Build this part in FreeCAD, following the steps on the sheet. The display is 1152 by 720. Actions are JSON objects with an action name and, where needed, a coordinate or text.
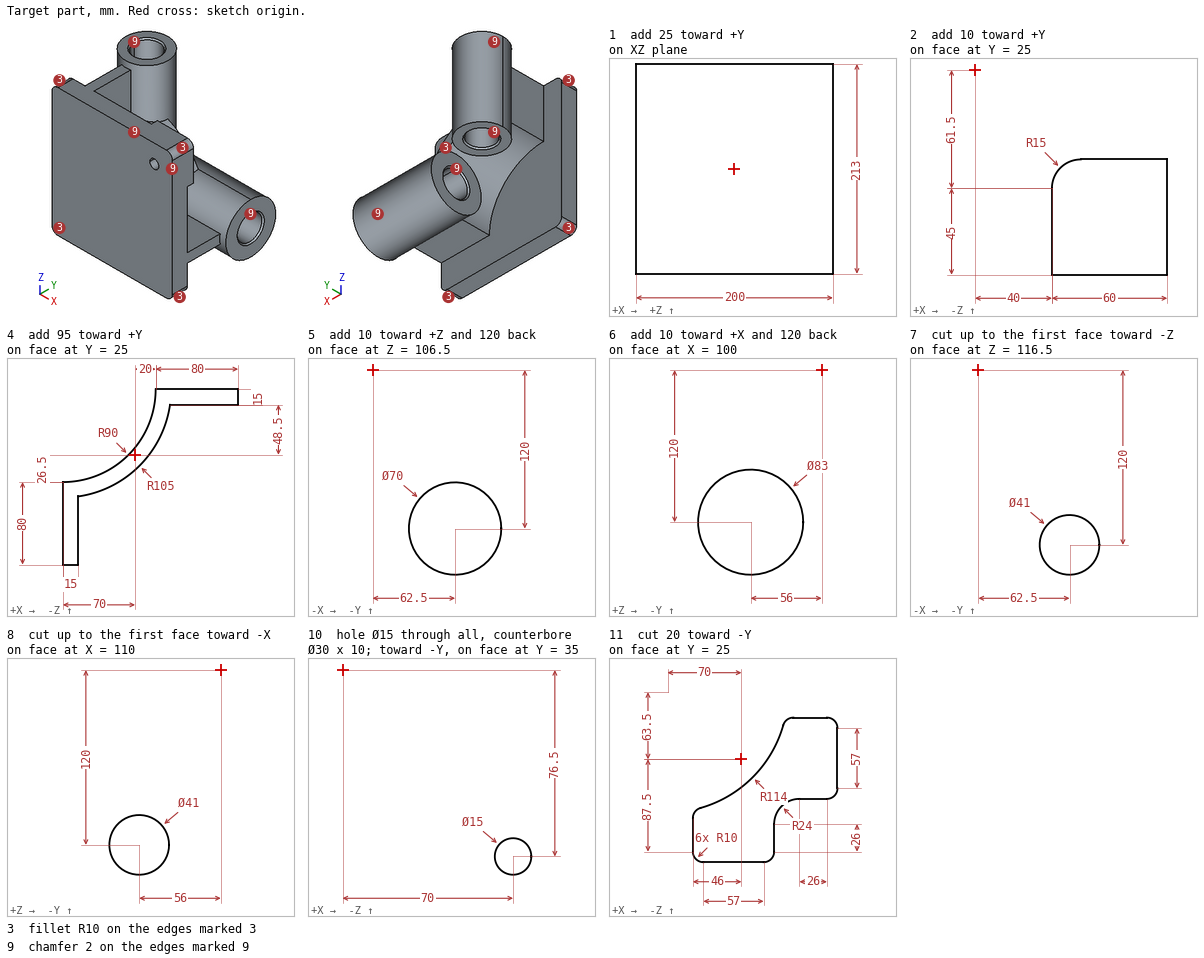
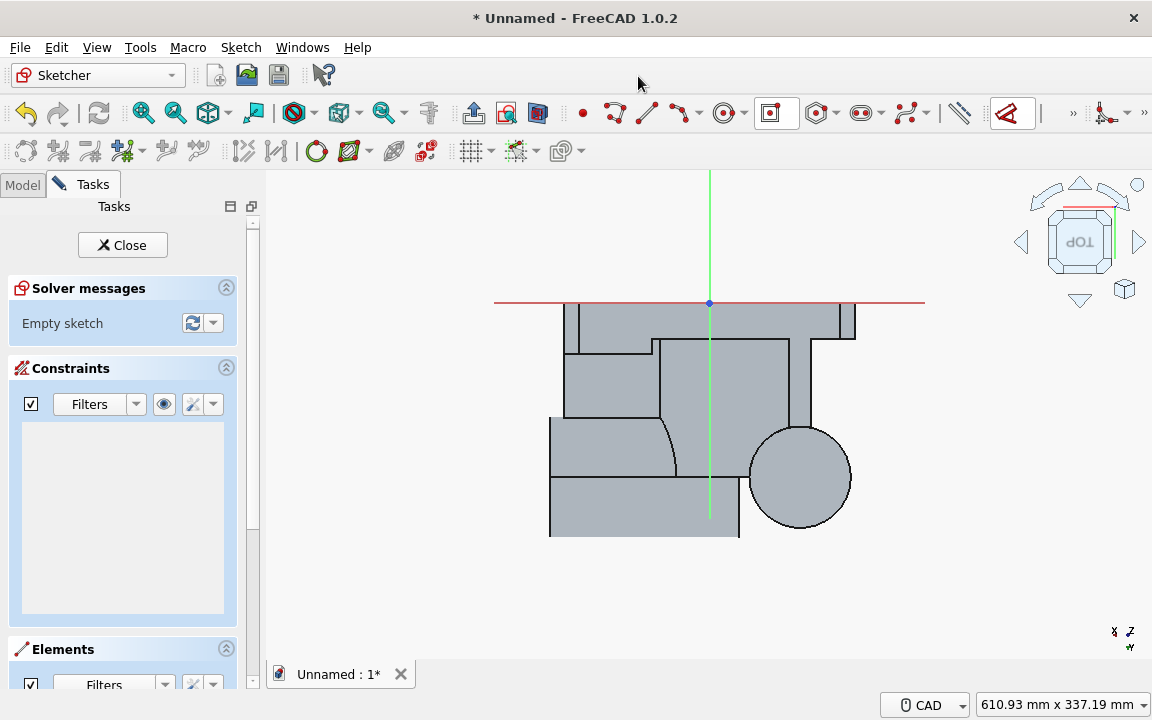
{"action": "scroll", "coordinate": [841, 493], "scroll_direction": "up", "scroll_amount": 8}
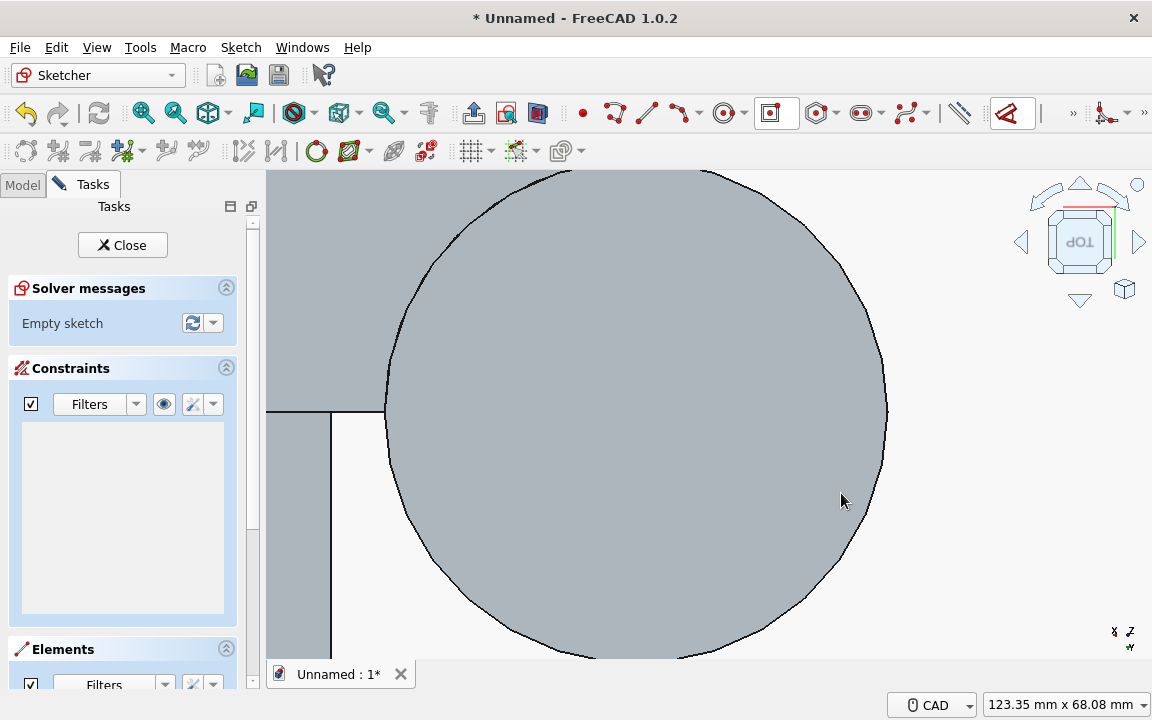
{"action": "left_click", "coordinate": [724, 114]}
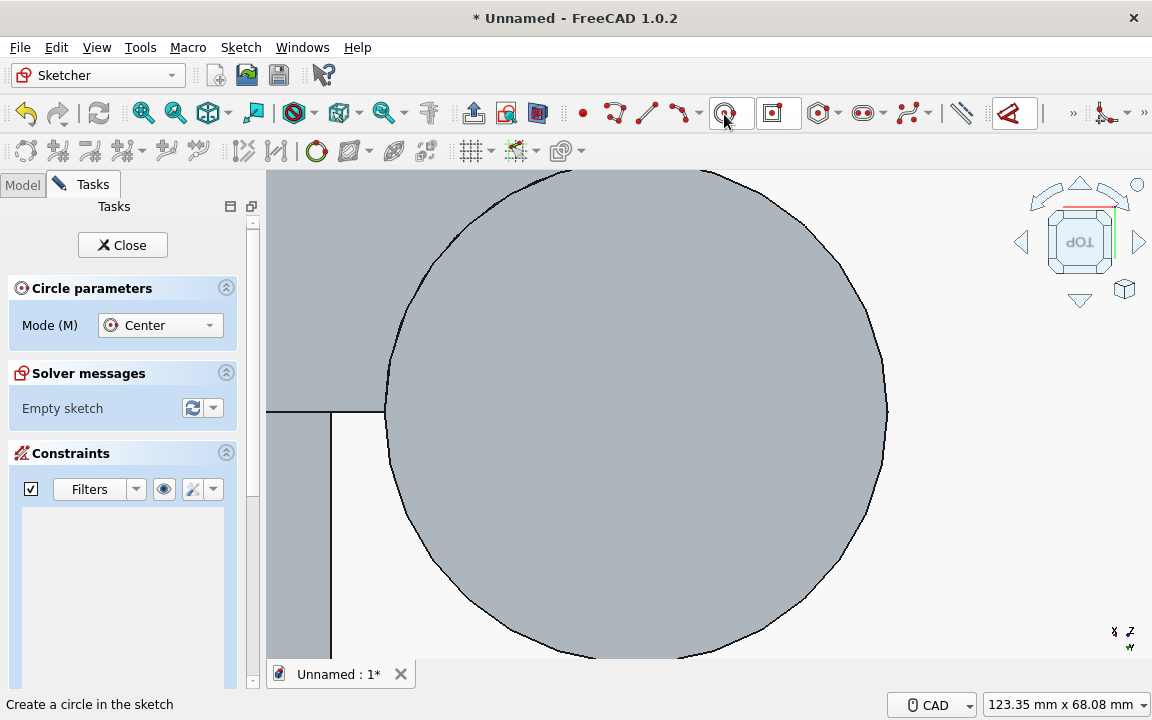
{"action": "left_click", "coordinate": [636, 412]}
{"action": "mouse_move", "coordinate": [740, 308]}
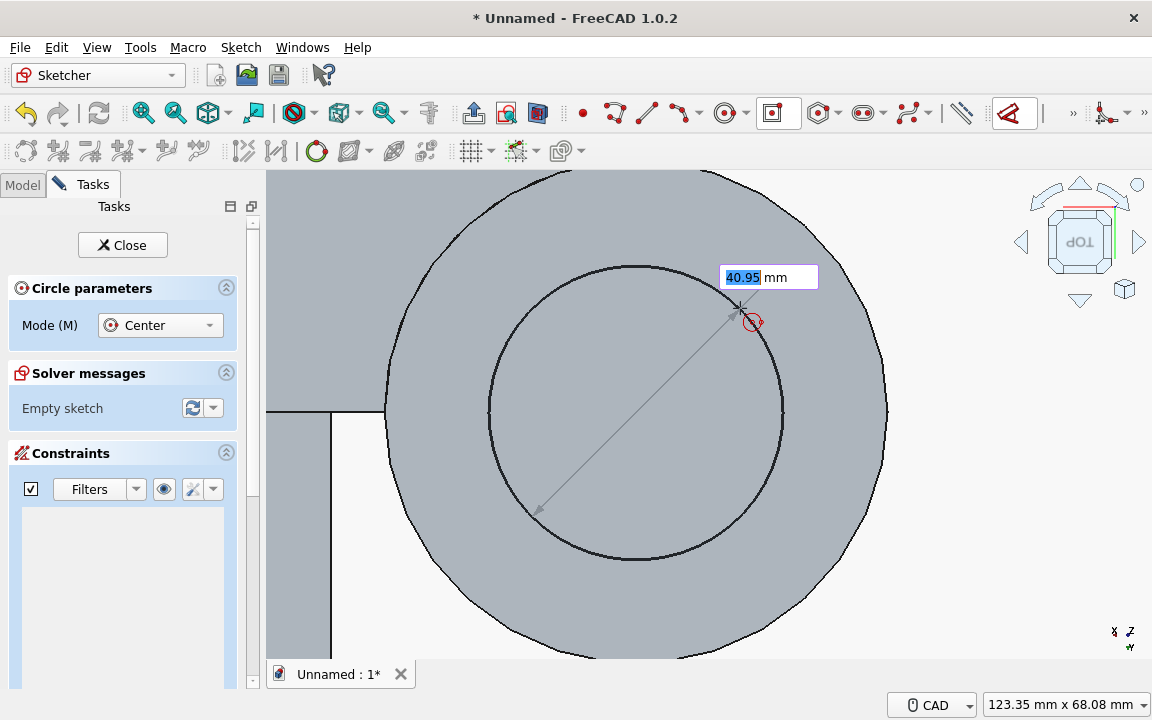
{"action": "type", "text": "41"}
{"action": "key", "text": "Return"}
{"action": "key", "text": "Escape"}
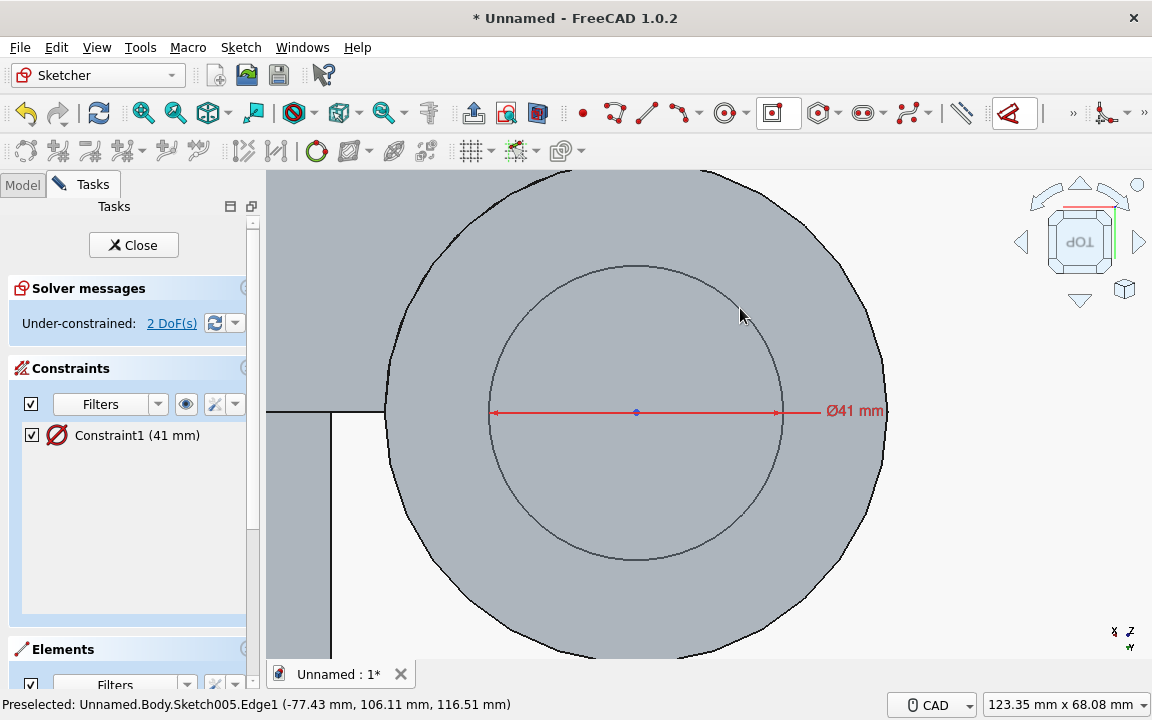
{"action": "left_click", "coordinate": [636, 413]}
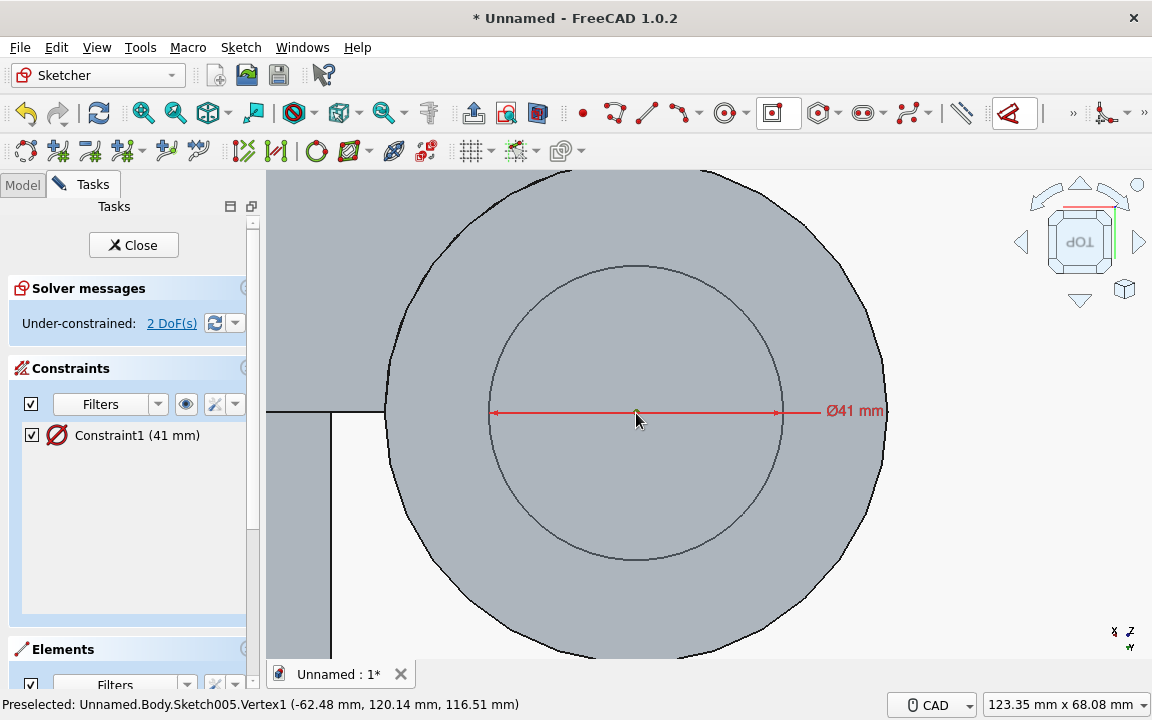
{"action": "key", "text": "i"}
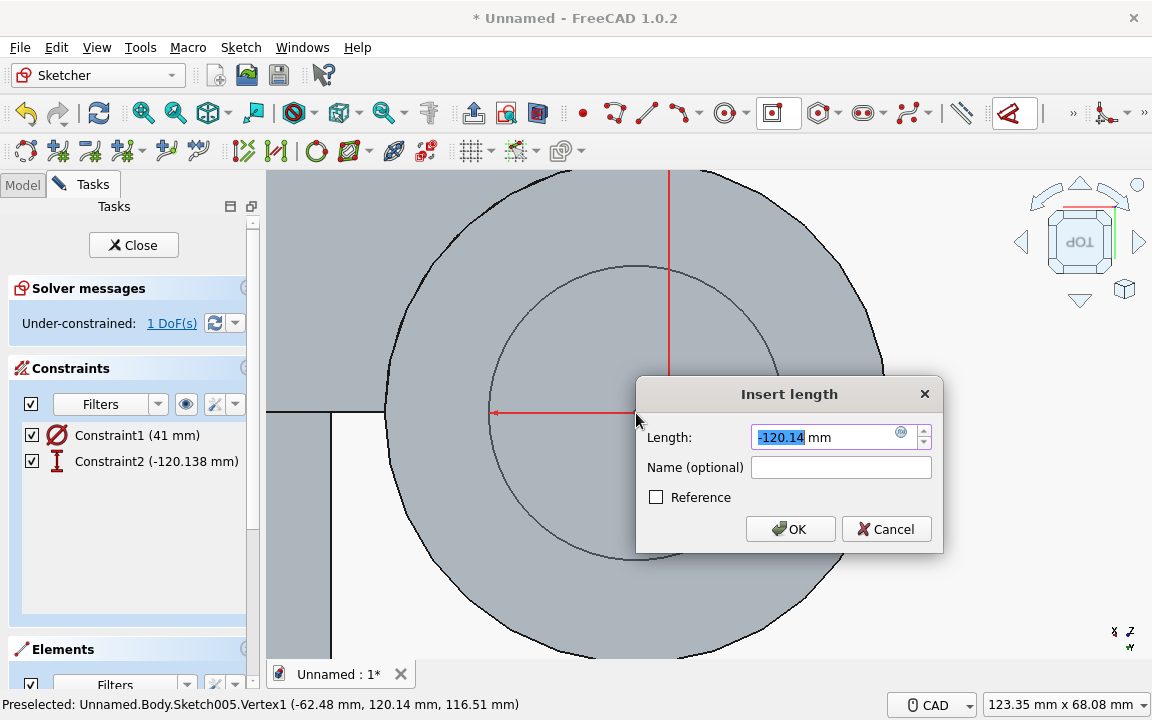
{"action": "type", "text": "-120"}
{"action": "key", "text": "Return"}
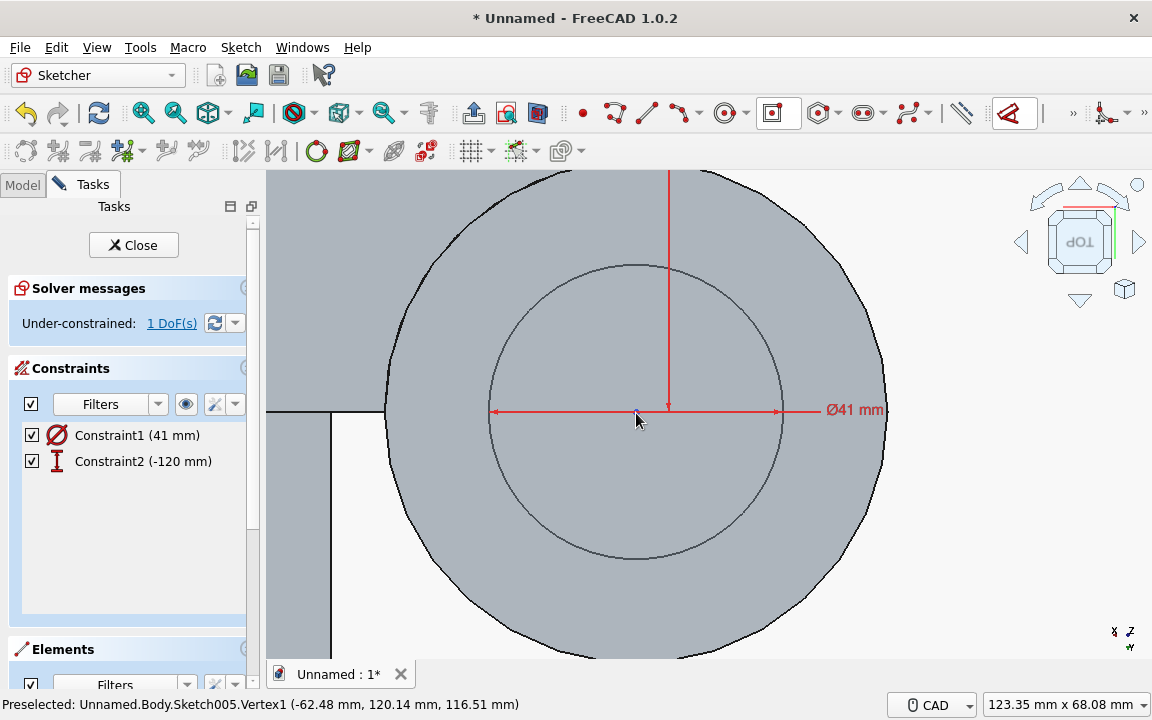
{"action": "left_click", "coordinate": [636, 412]}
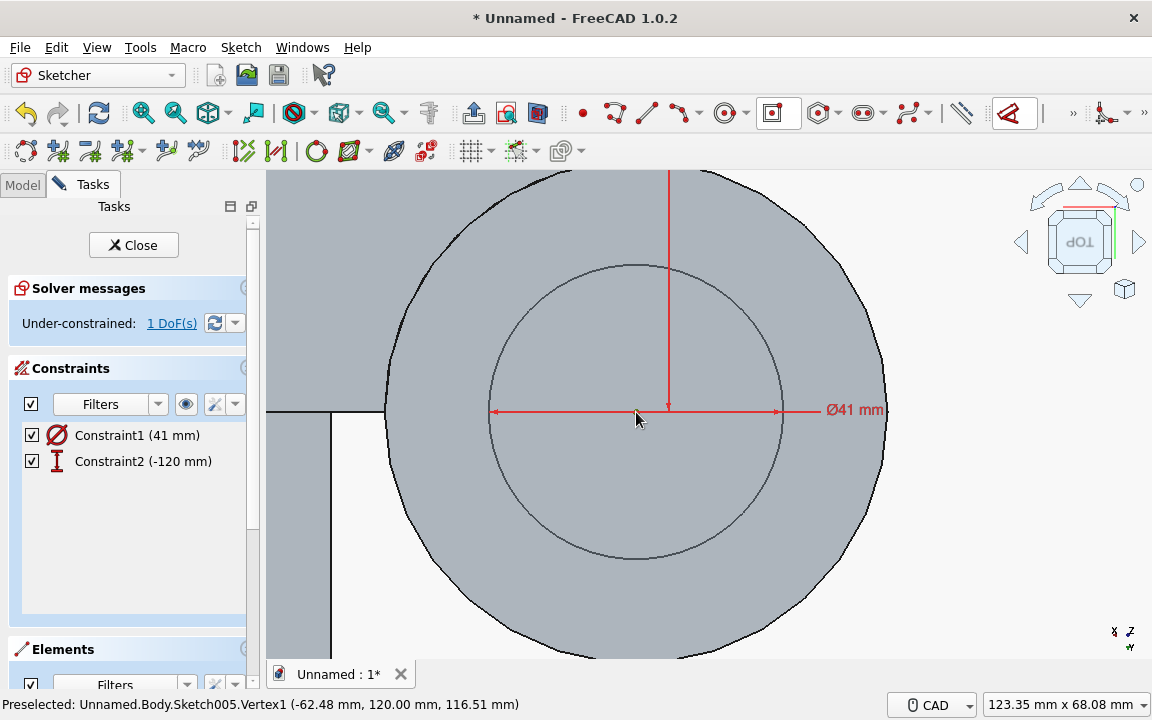
{"action": "left_click", "coordinate": [1032, 114]}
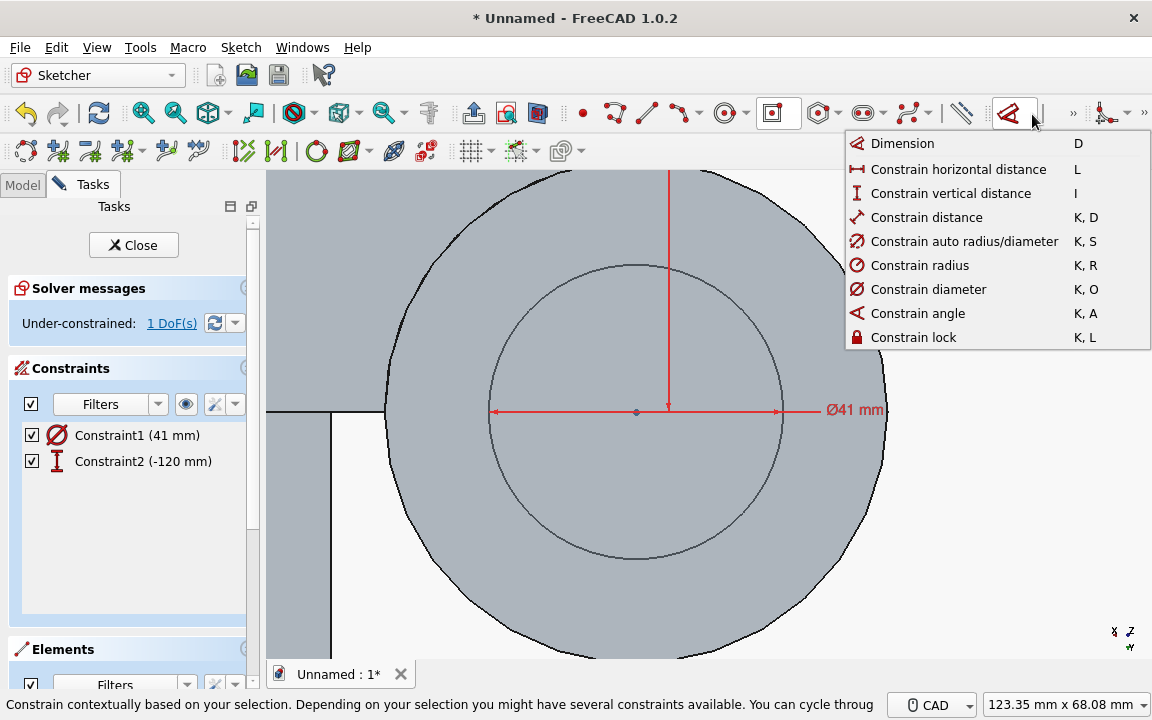
{"action": "left_click", "coordinate": [998, 169]}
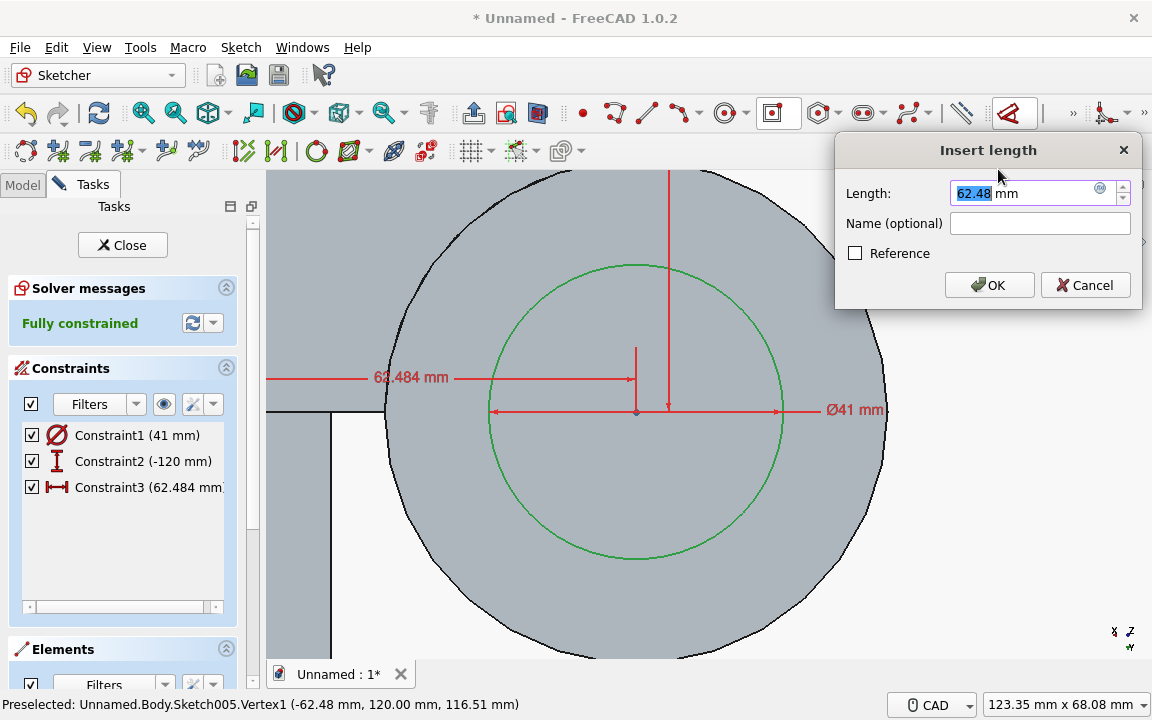
{"action": "type", "text": "62.5"}
{"action": "key", "text": "Return"}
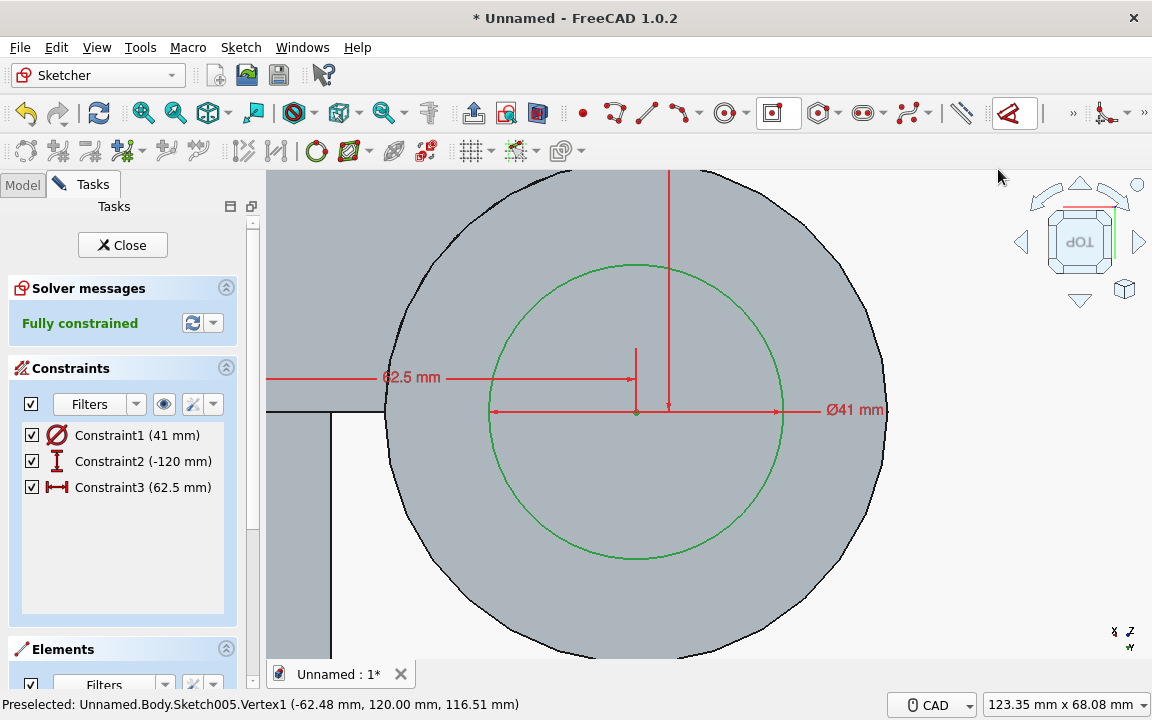
{"action": "left_click", "coordinate": [123, 245]}